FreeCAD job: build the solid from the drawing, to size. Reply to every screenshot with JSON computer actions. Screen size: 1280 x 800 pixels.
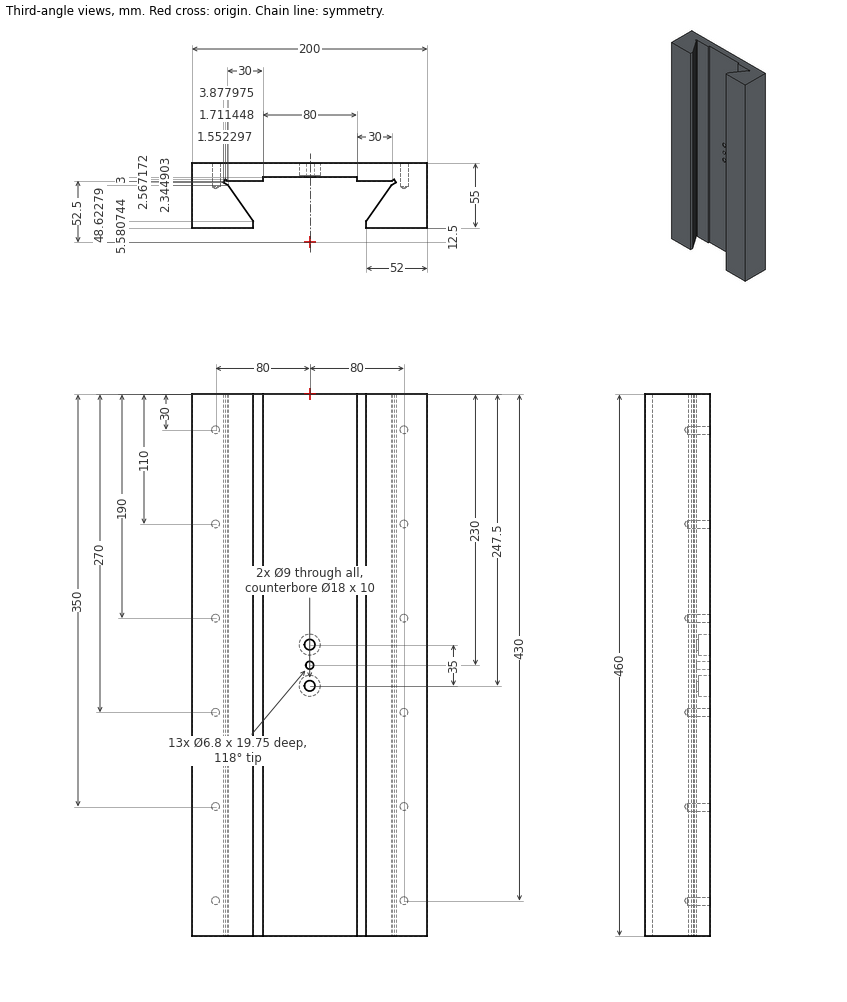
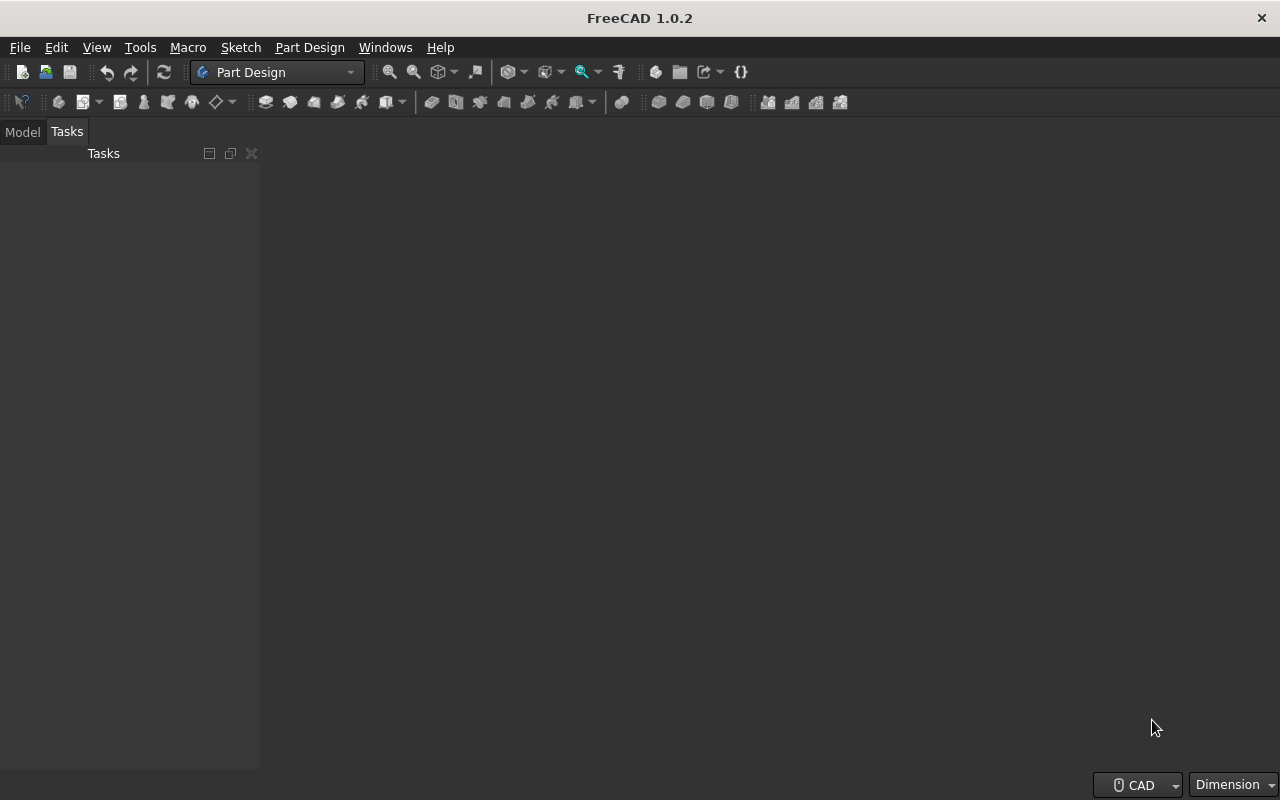
{"action": "left_click", "coordinate": [22, 72]}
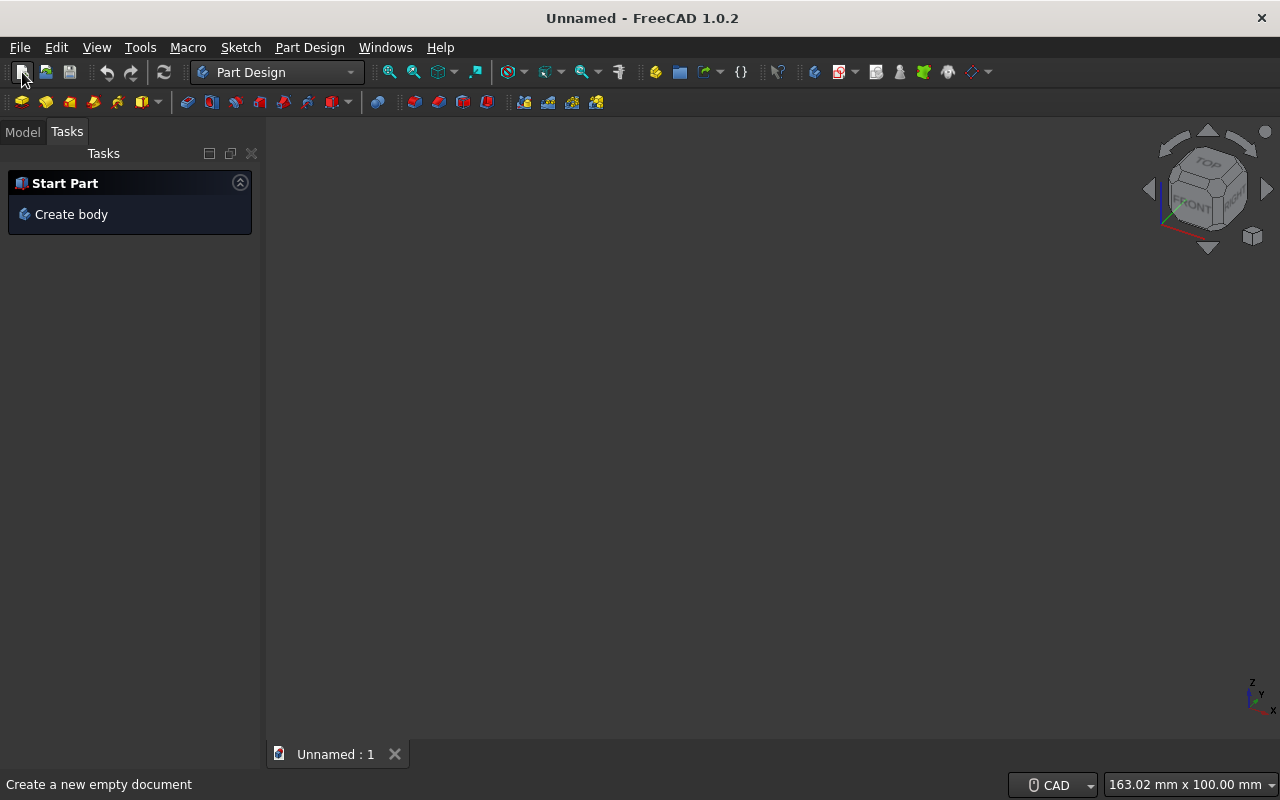
{"action": "left_click", "coordinate": [840, 72]}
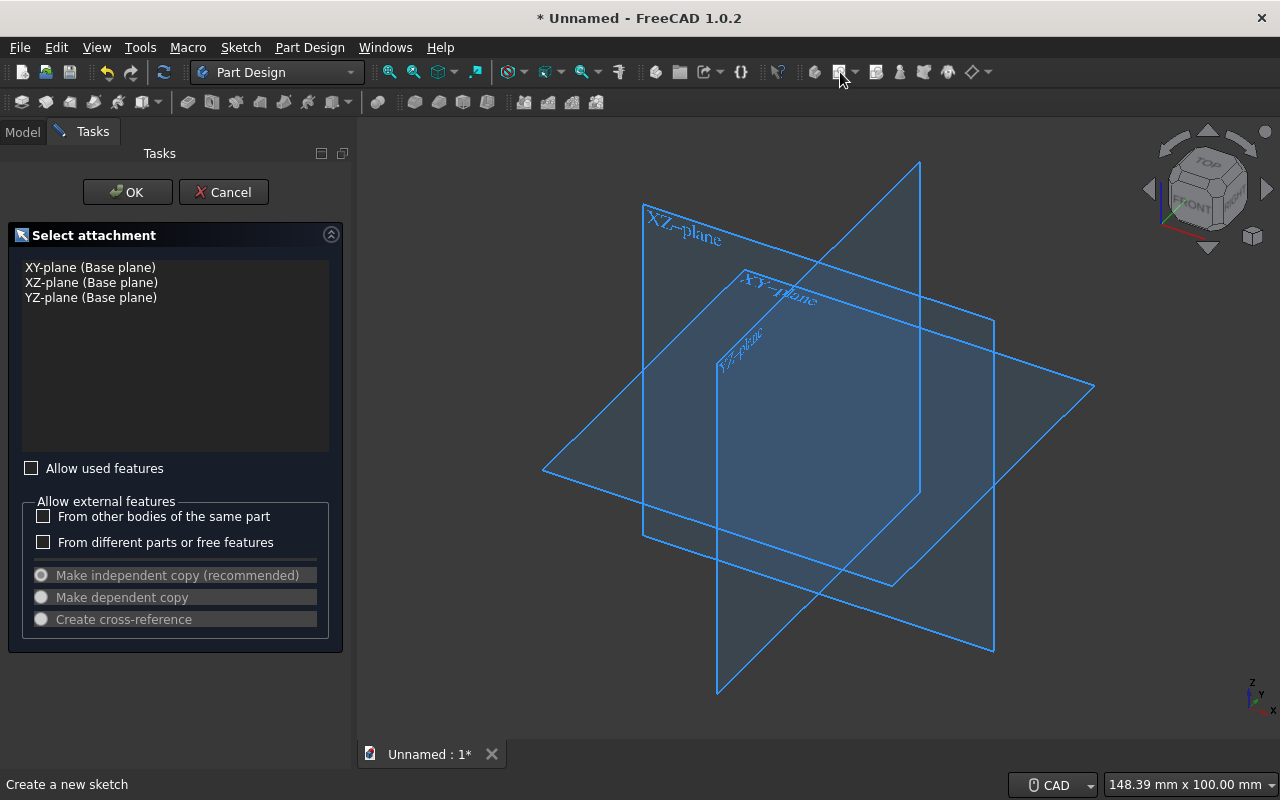
{"action": "left_click", "coordinate": [82, 268]}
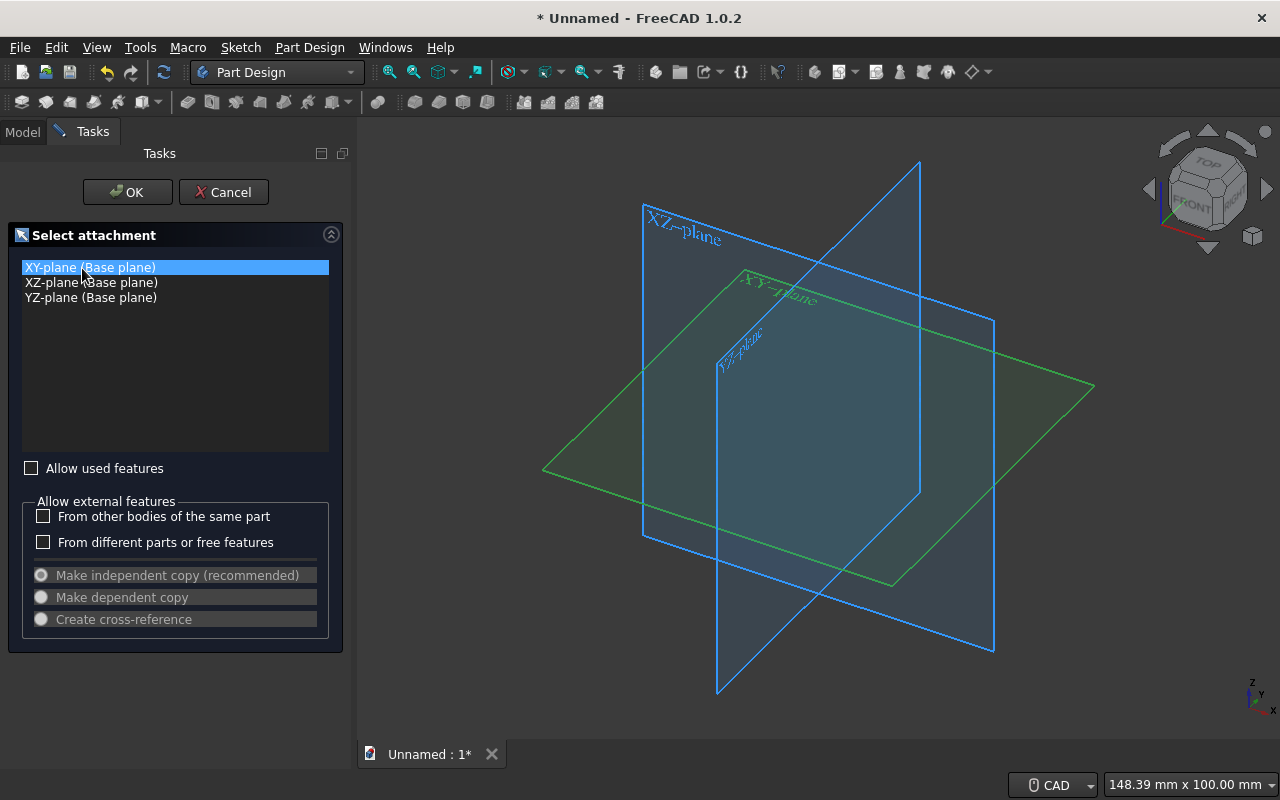
{"action": "left_click", "coordinate": [128, 192]}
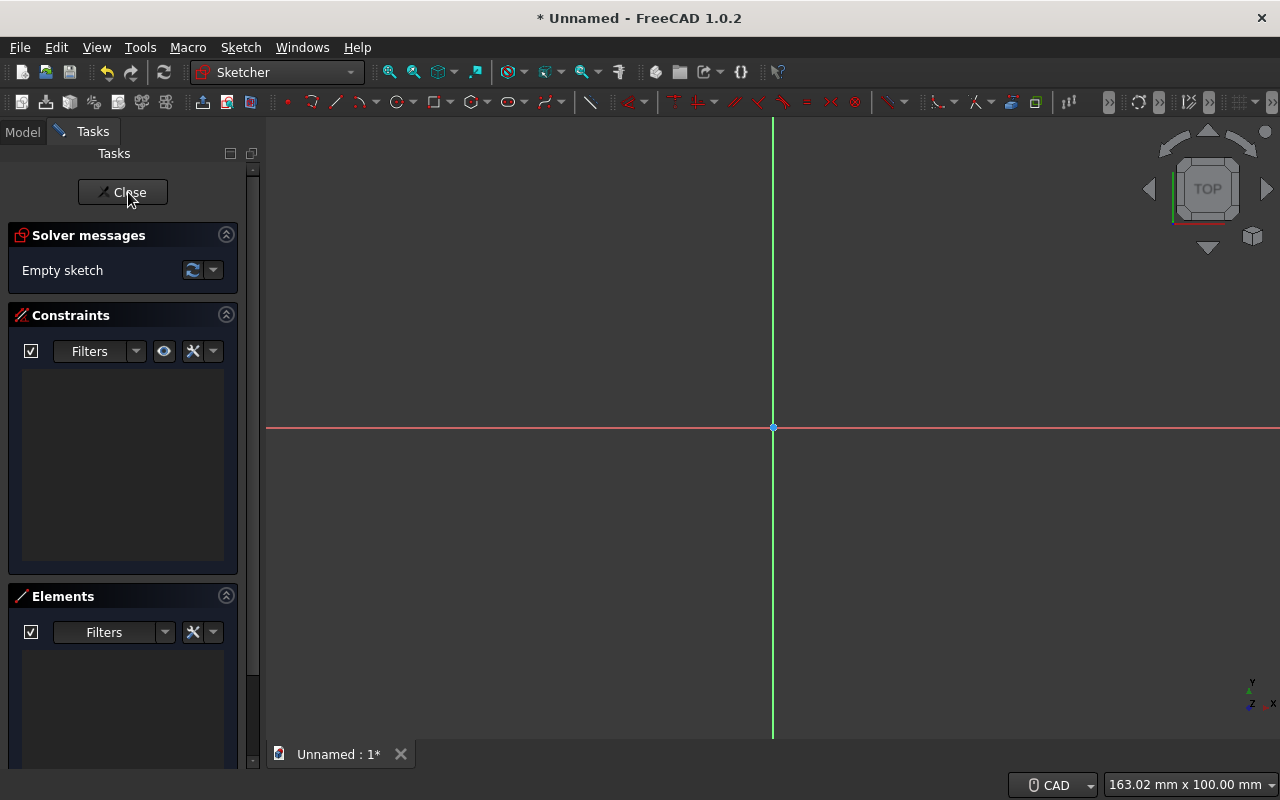
{"action": "scroll", "coordinate": [649, 599], "scroll_direction": "down", "scroll_amount": 4}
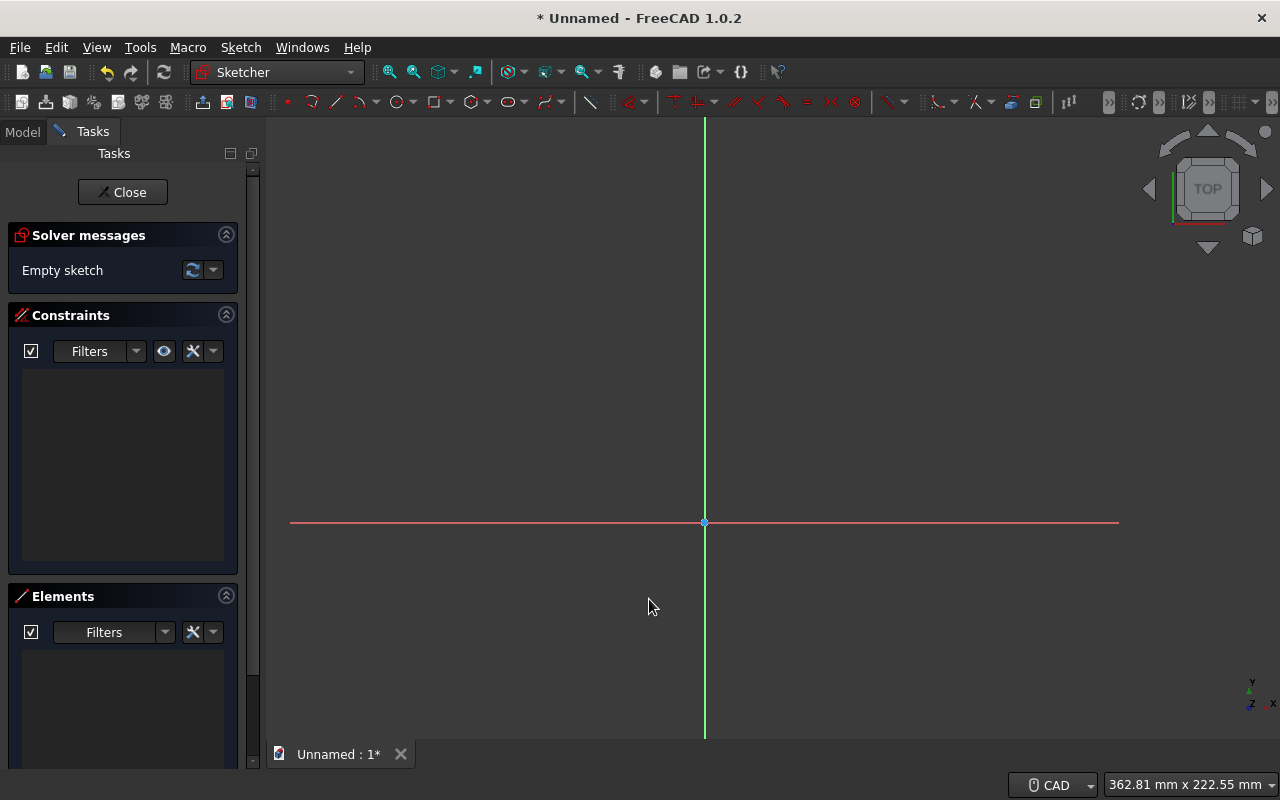
{"action": "left_click", "coordinate": [312, 102]}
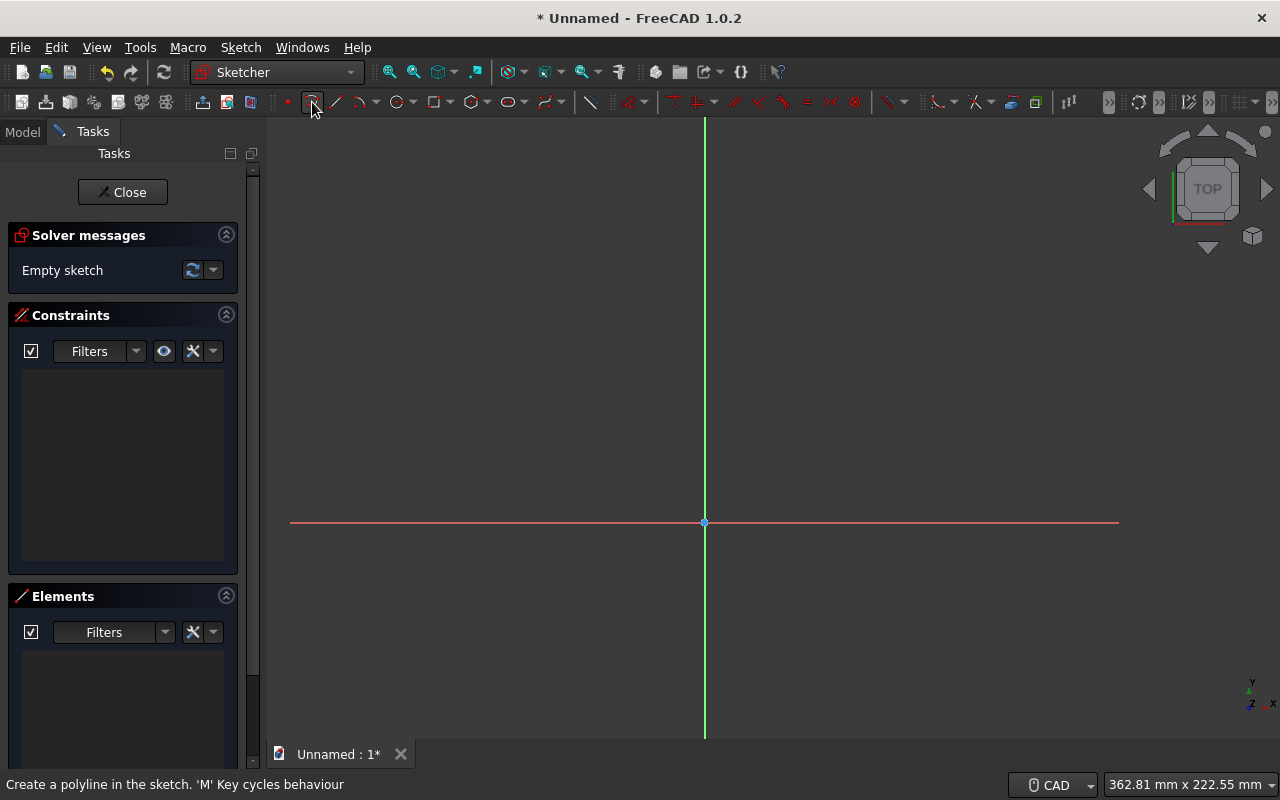
{"action": "left_click", "coordinate": [839, 488]}
{"action": "left_click", "coordinate": [984, 488]}
{"action": "left_click", "coordinate": [984, 334]}
{"action": "left_click", "coordinate": [425, 334]}
{"action": "left_click", "coordinate": [425, 488]}
{"action": "left_click", "coordinate": [571, 488]}
{"action": "left_click", "coordinate": [571, 472]}
{"action": "left_click", "coordinate": [511, 387]}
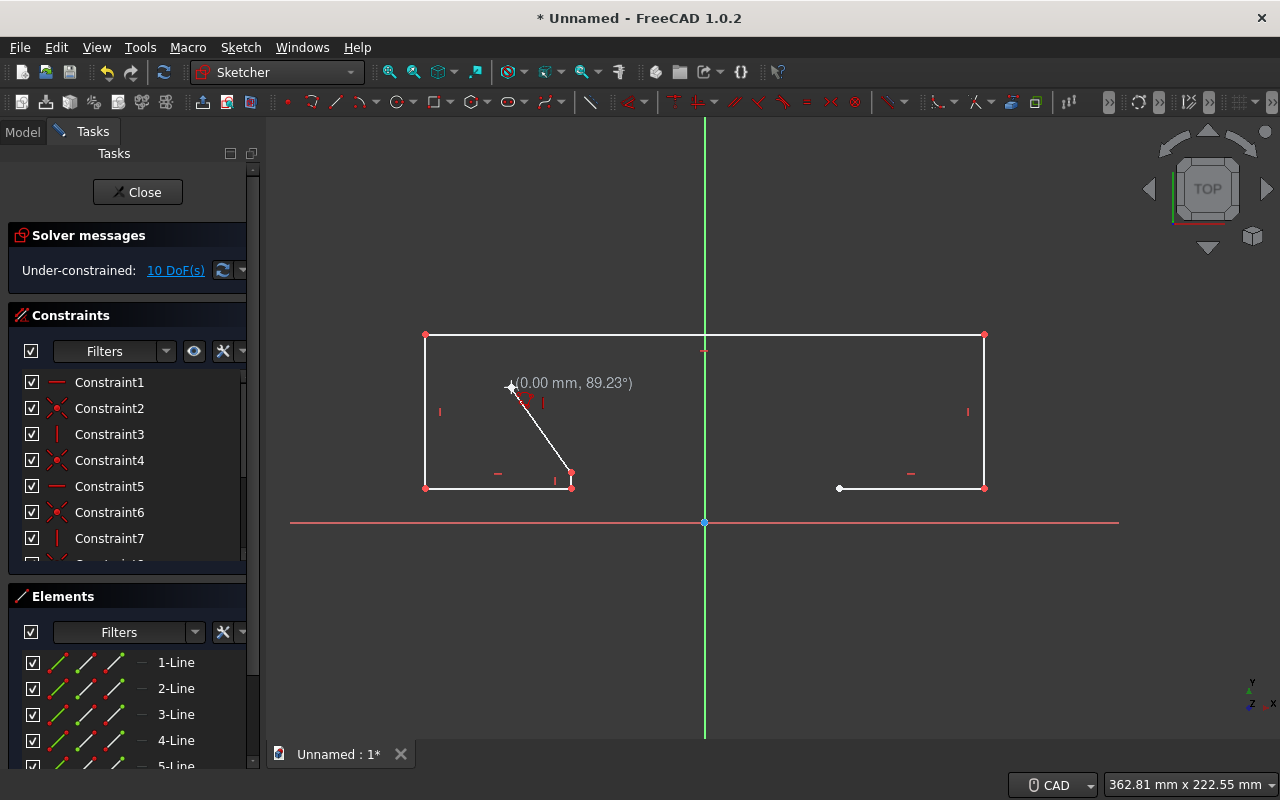
{"action": "scroll", "coordinate": [500, 380], "scroll_direction": "up", "scroll_amount": 2}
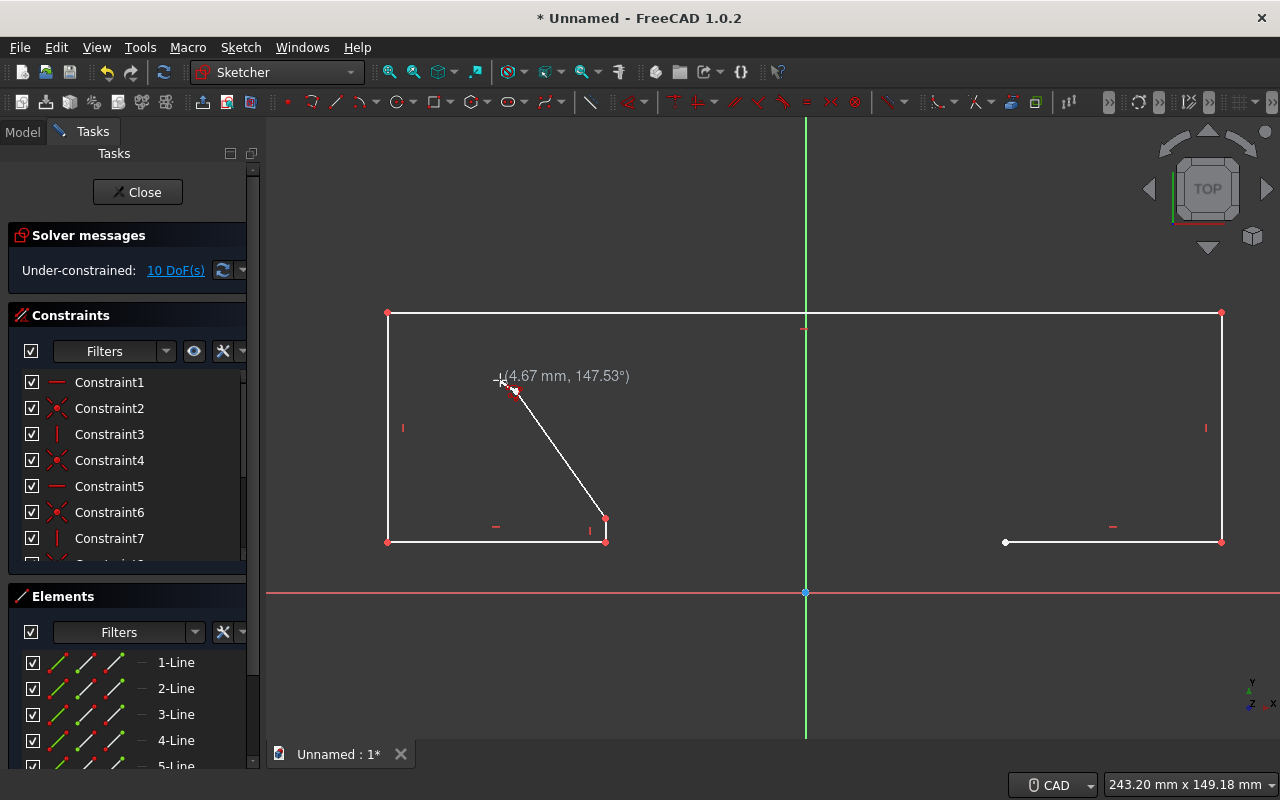
{"action": "left_click", "coordinate": [500, 380]}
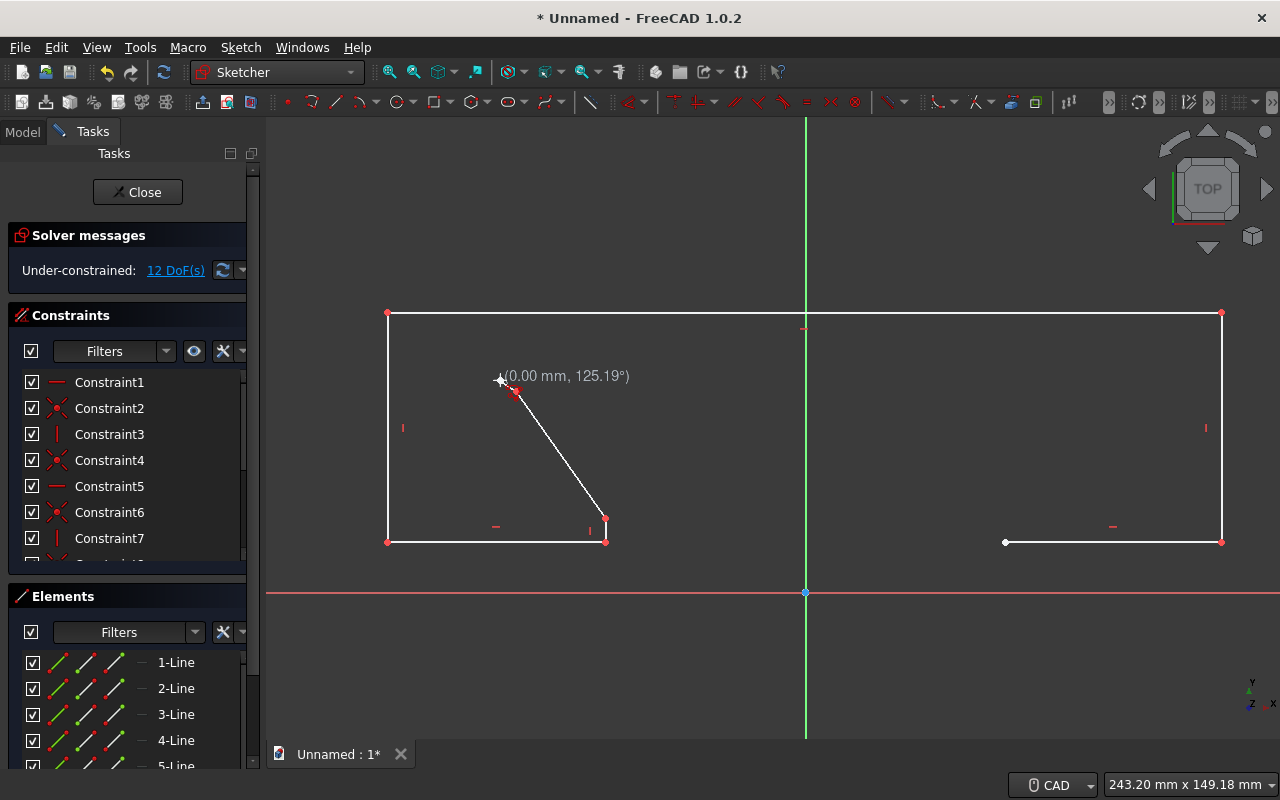
{"action": "scroll", "coordinate": [507, 369], "scroll_direction": "up", "scroll_amount": 2}